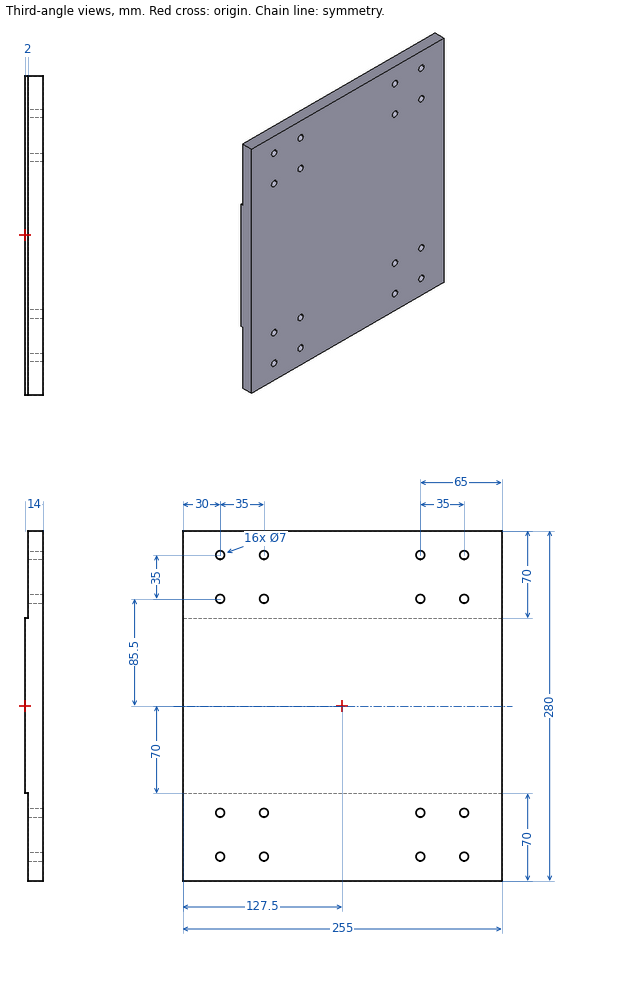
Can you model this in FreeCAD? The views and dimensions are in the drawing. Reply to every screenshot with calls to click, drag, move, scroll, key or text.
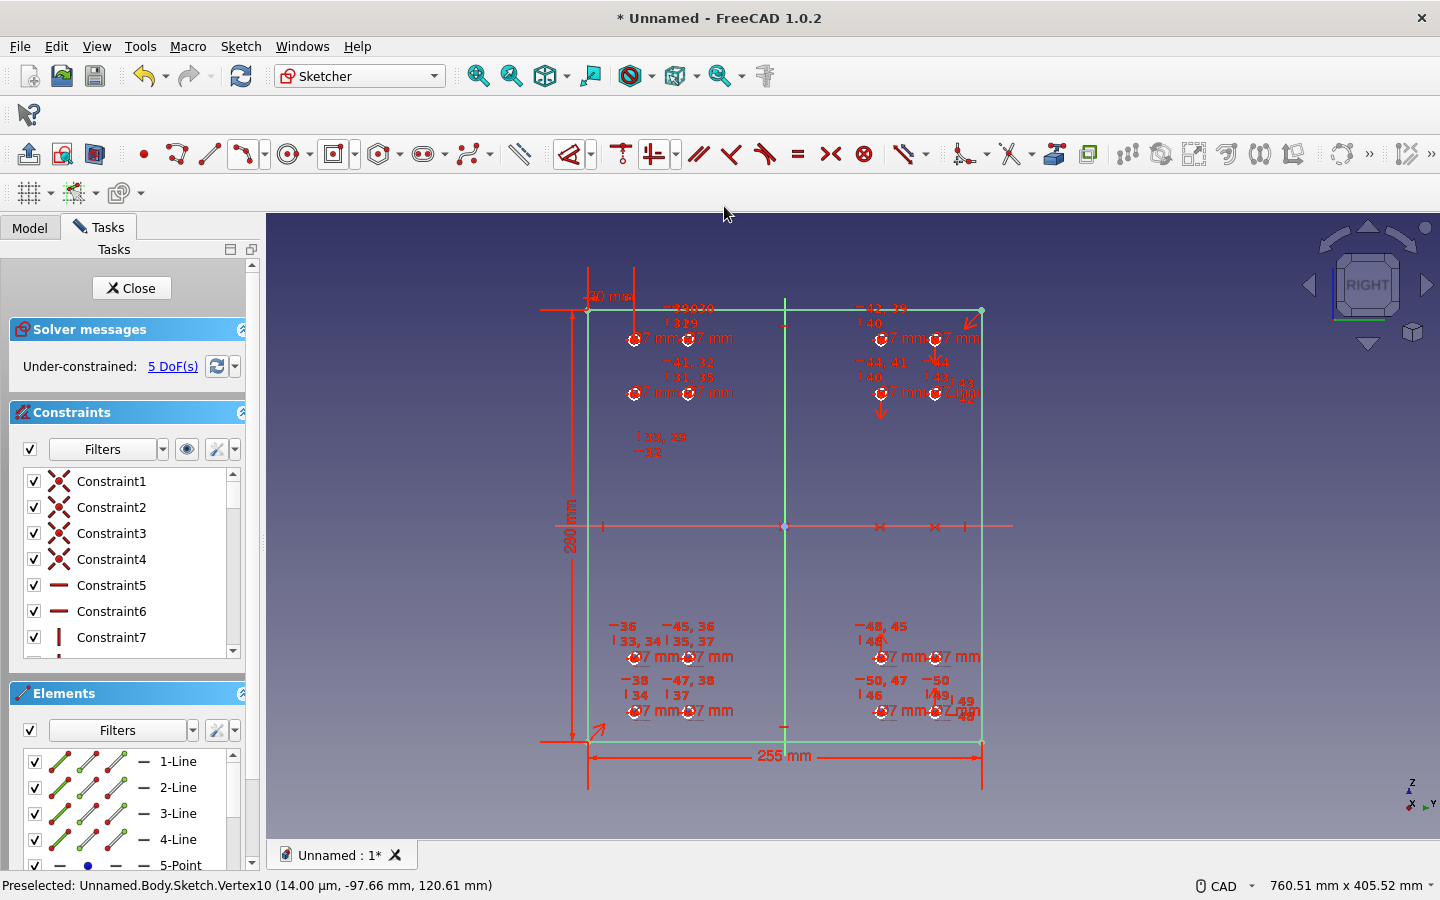
click(634, 340)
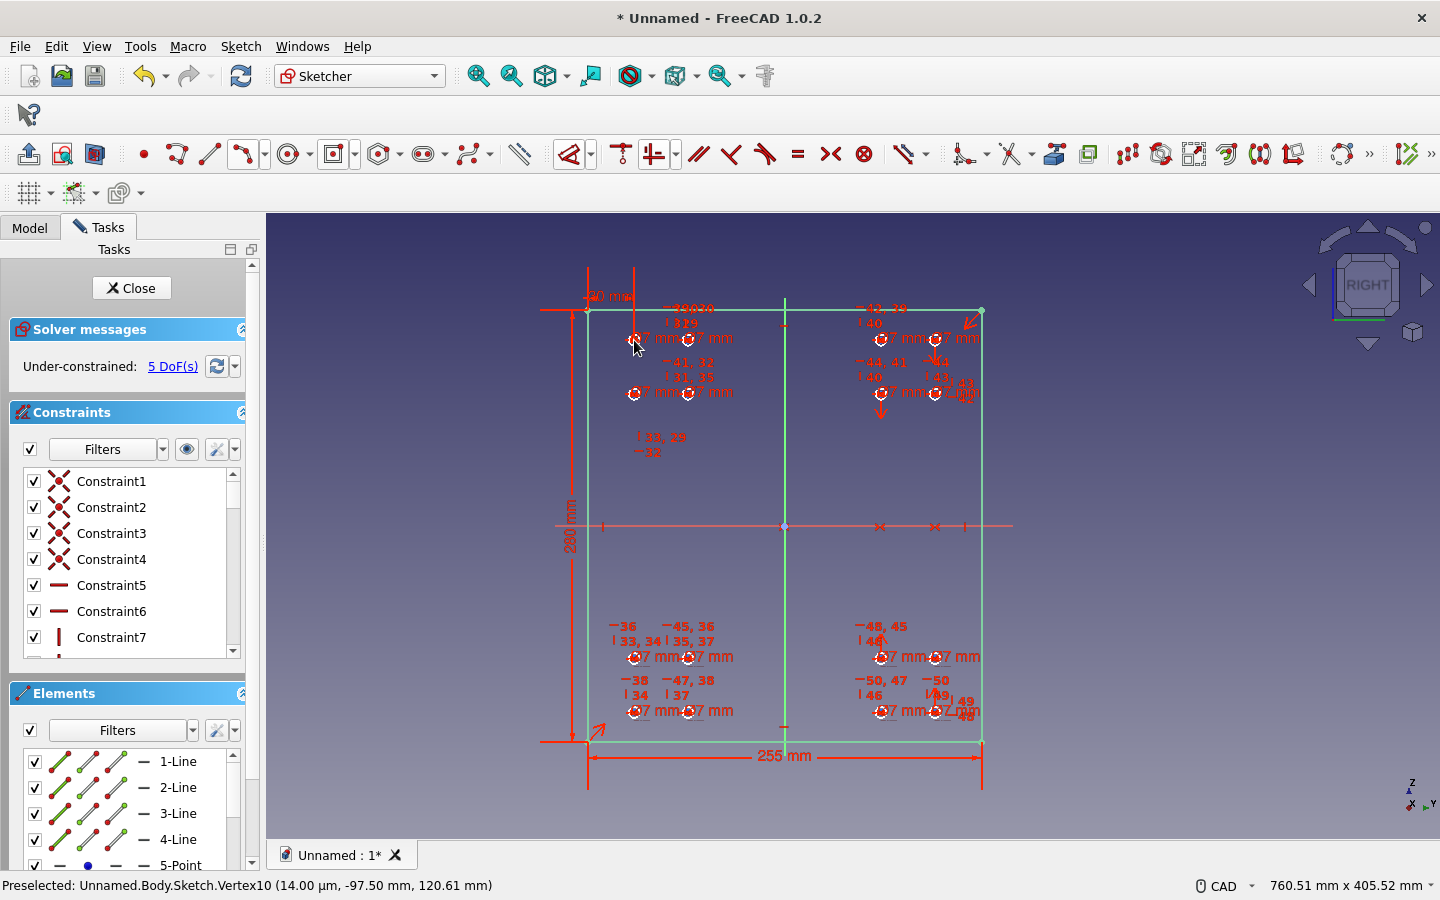
click(634, 394)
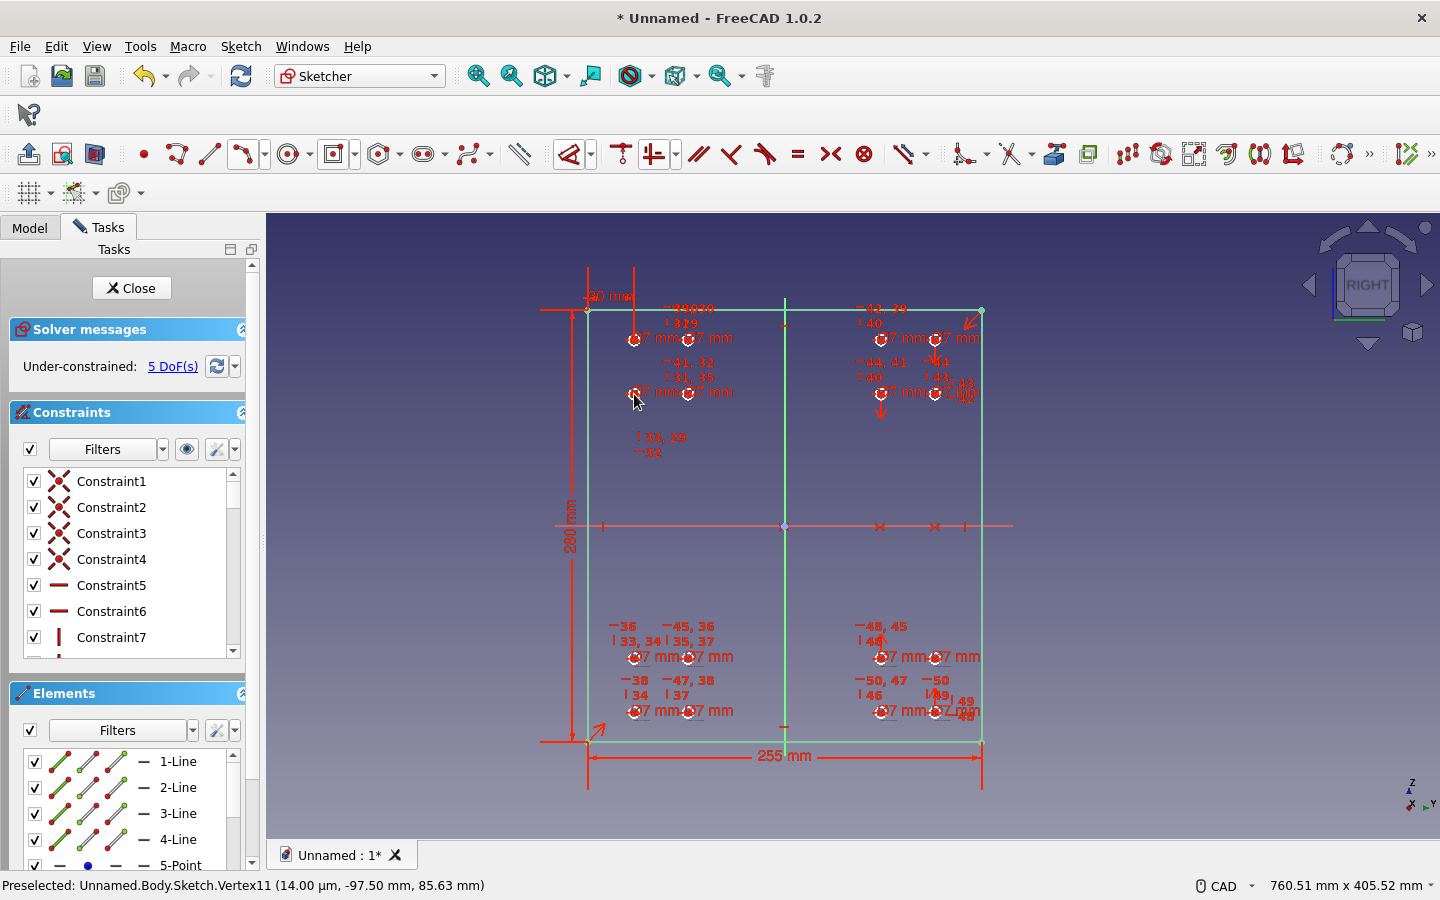
click(590, 154)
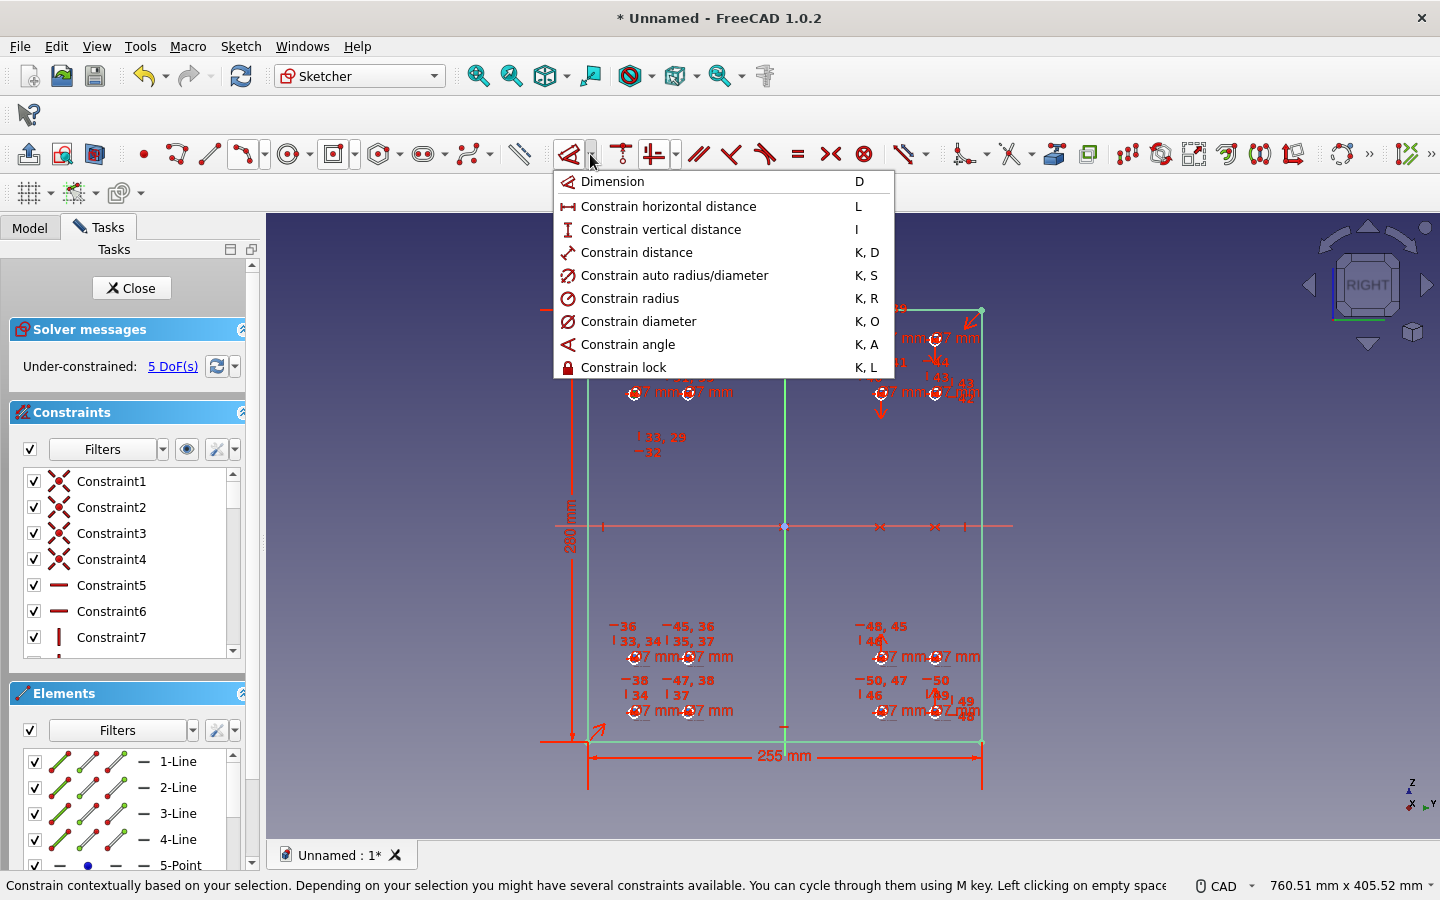
click(724, 230)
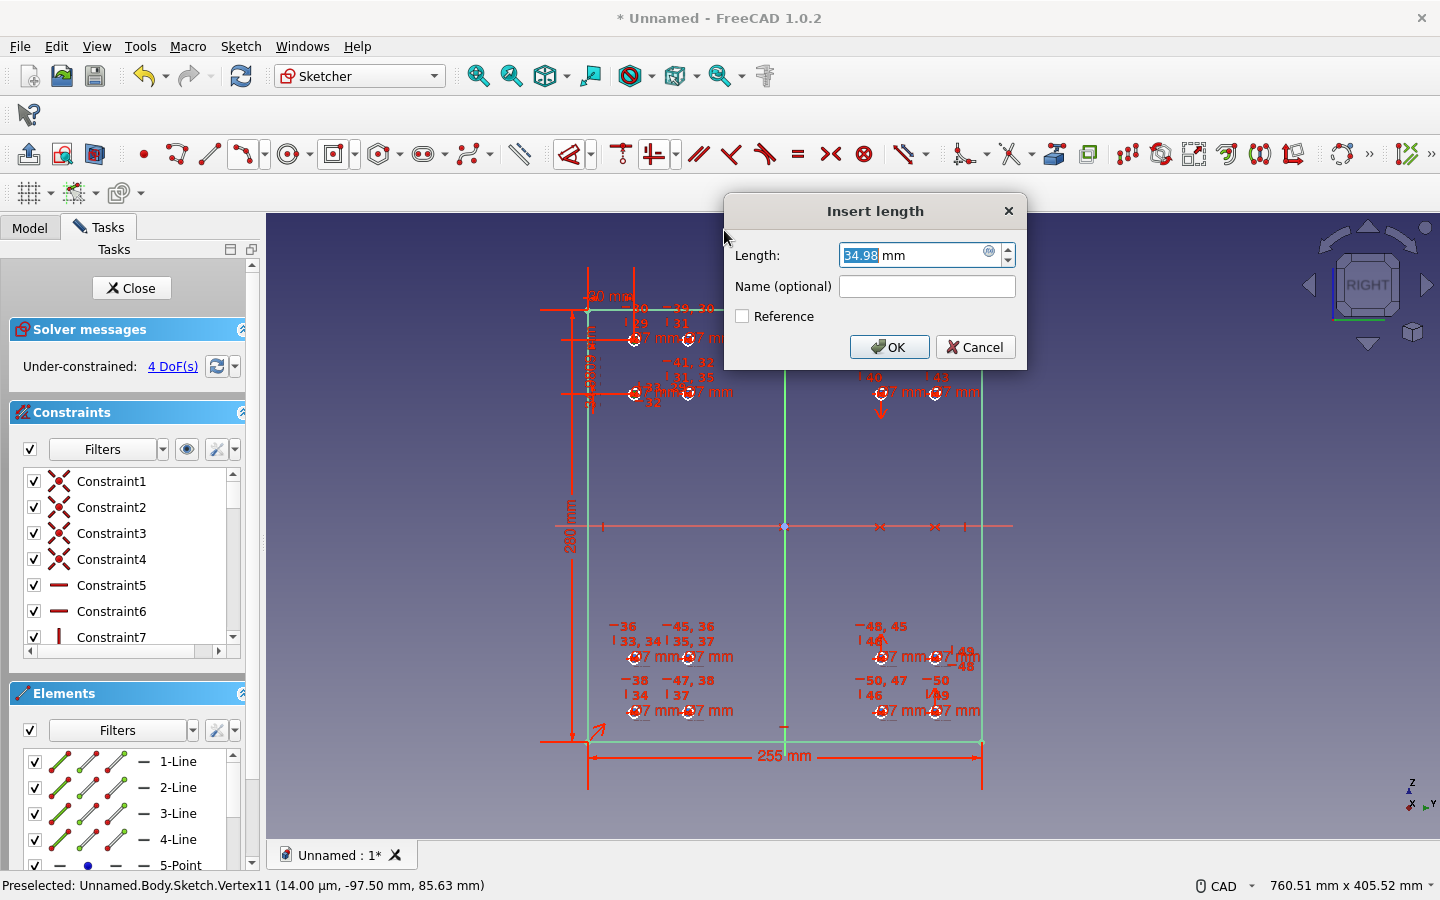
text(35)
key(Return)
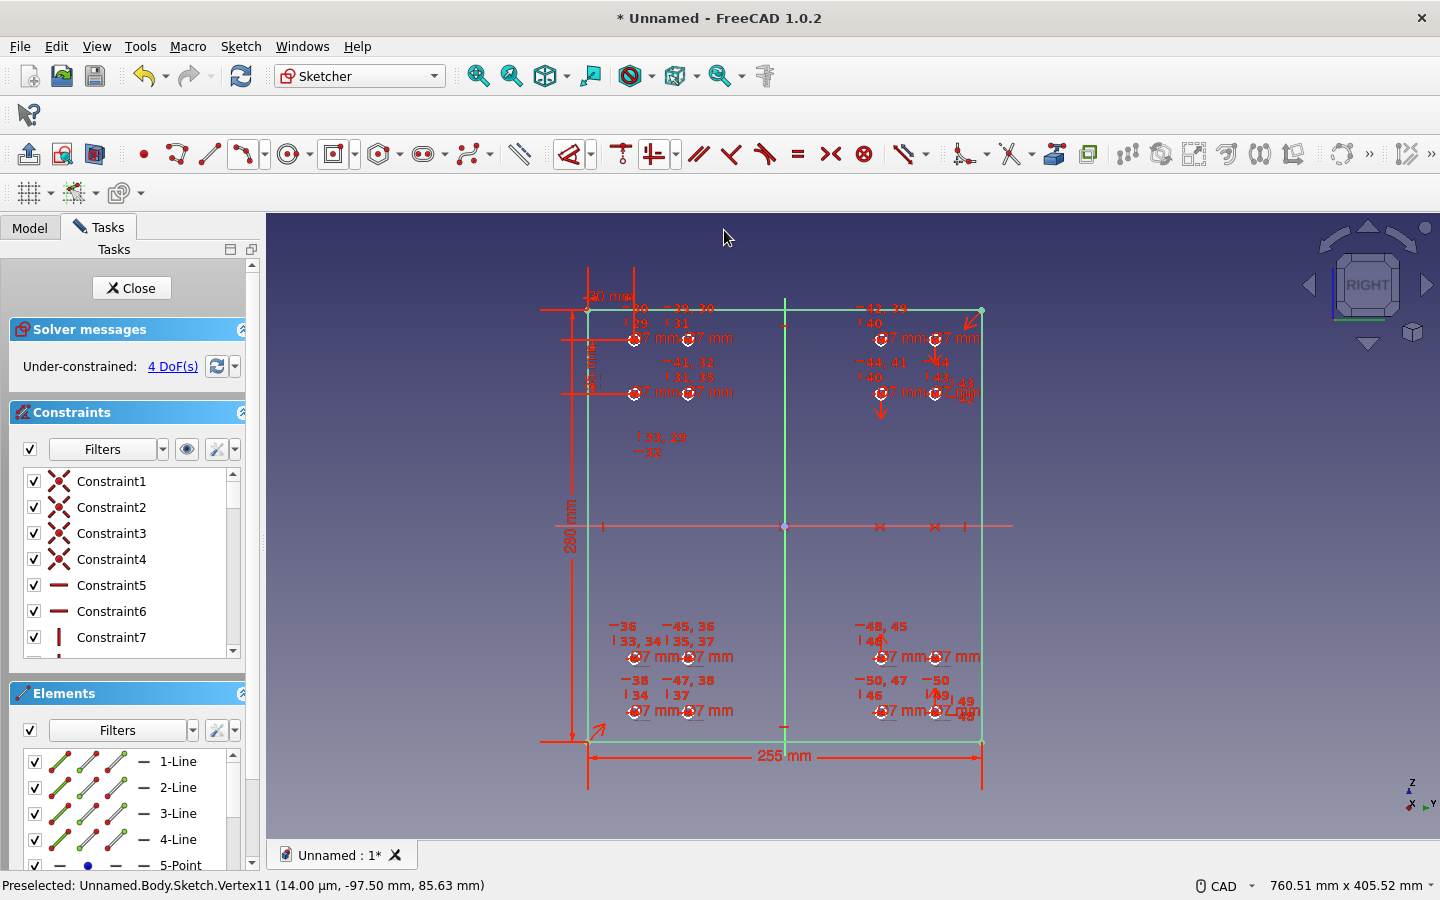
click(634, 340)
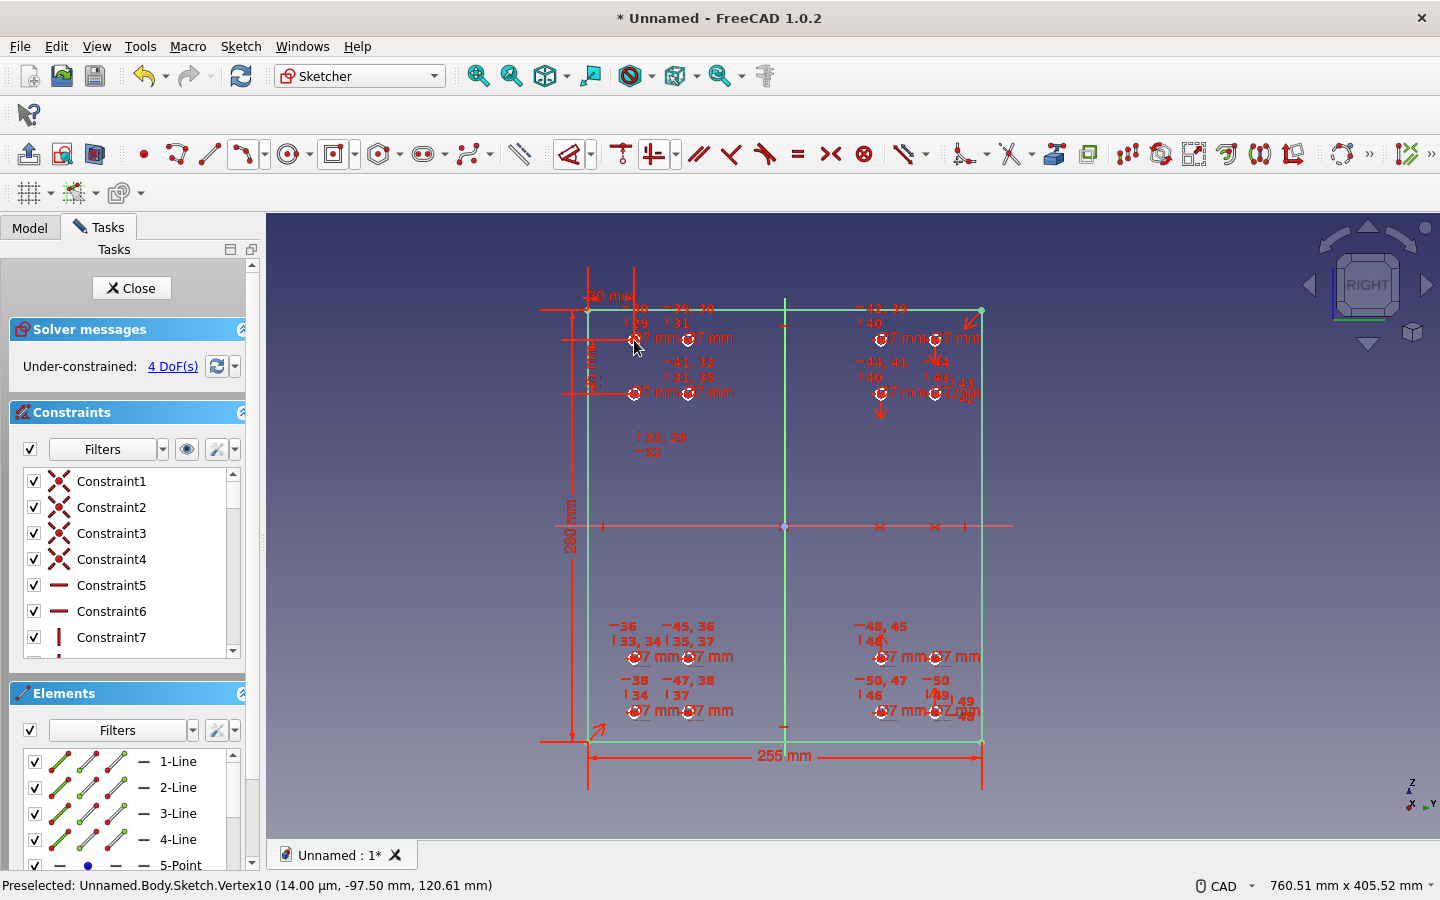
click(688, 340)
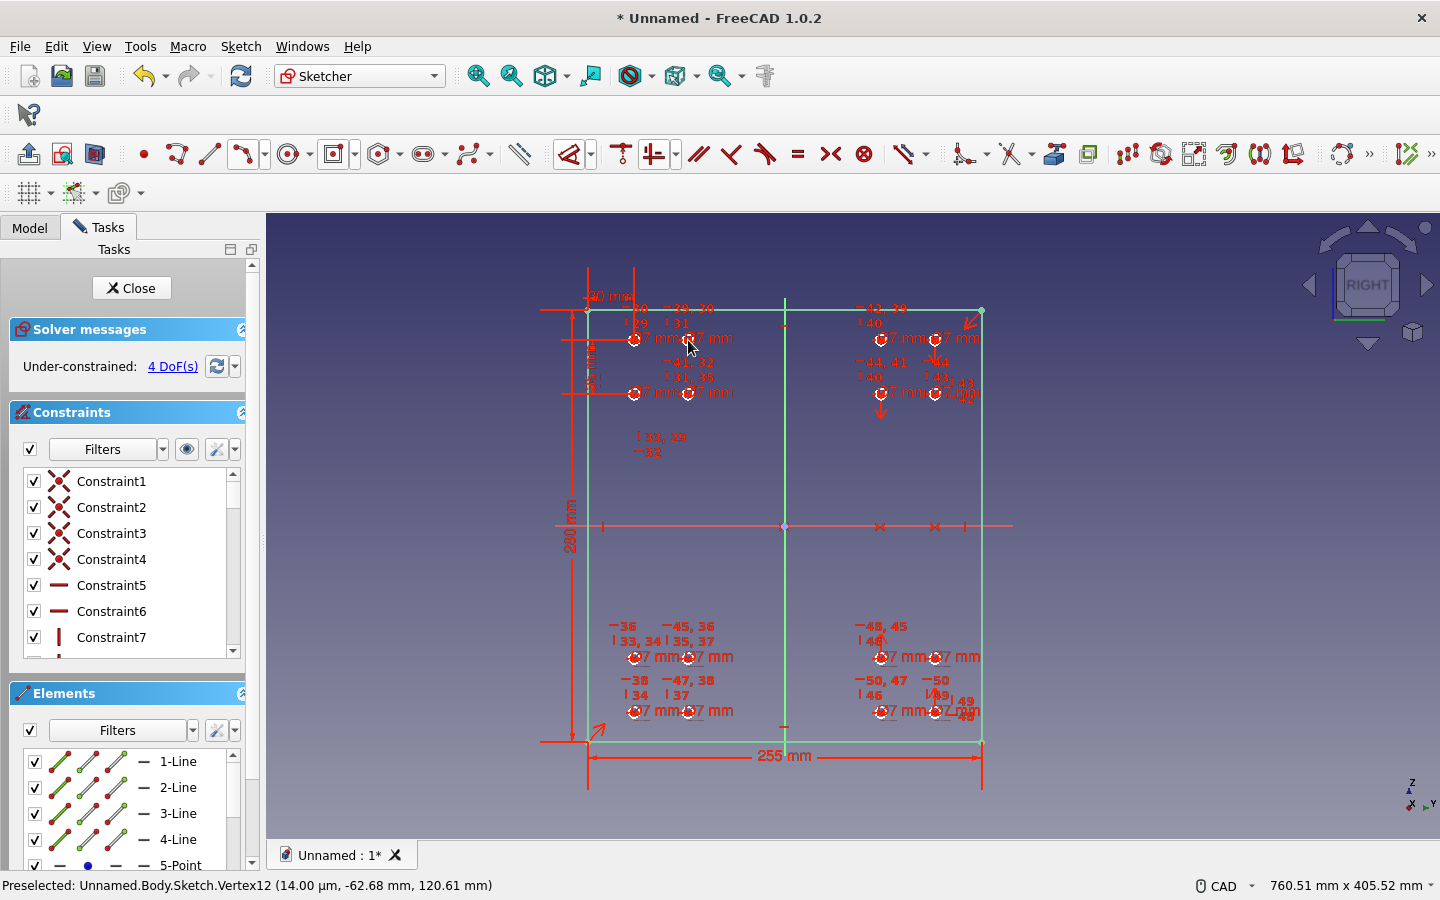
click(590, 154)